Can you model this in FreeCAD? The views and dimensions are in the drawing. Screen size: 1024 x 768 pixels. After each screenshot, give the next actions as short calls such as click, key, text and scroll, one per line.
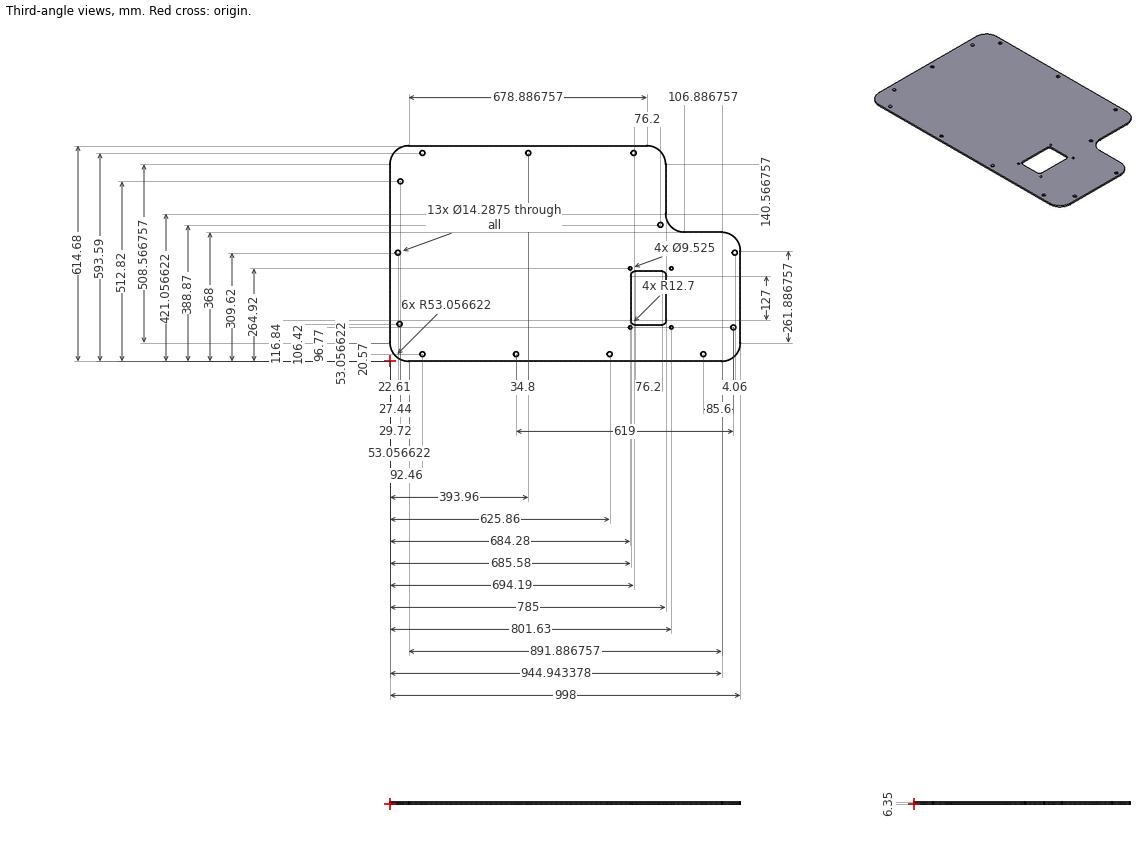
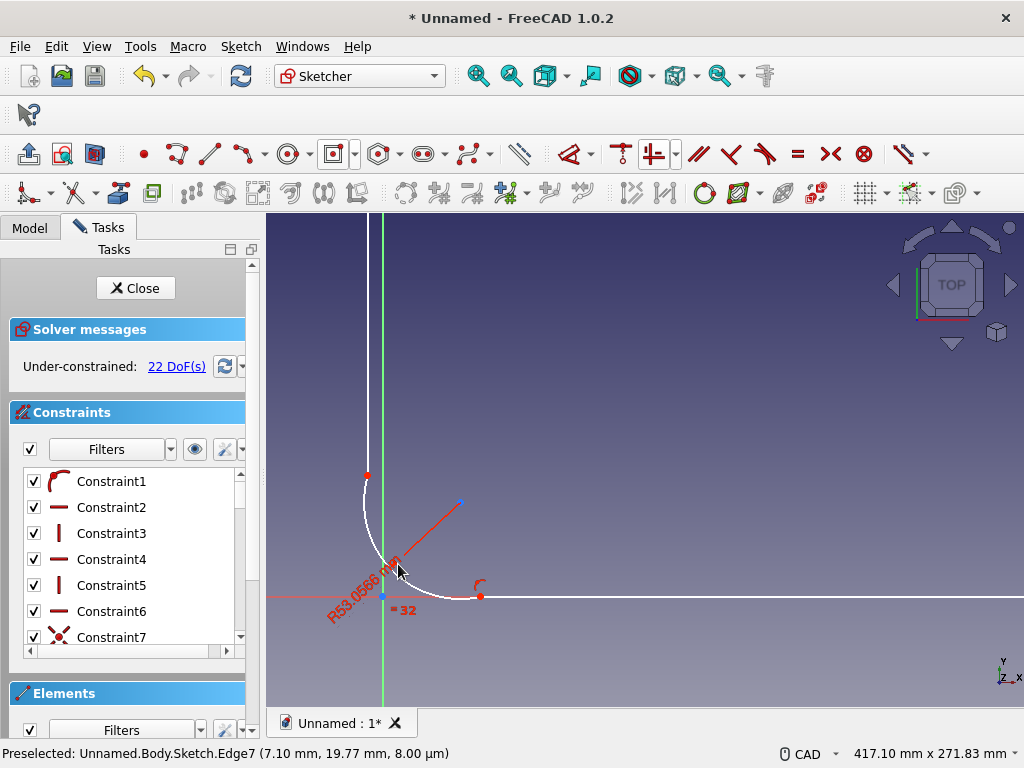
scroll(396, 567, down, 8)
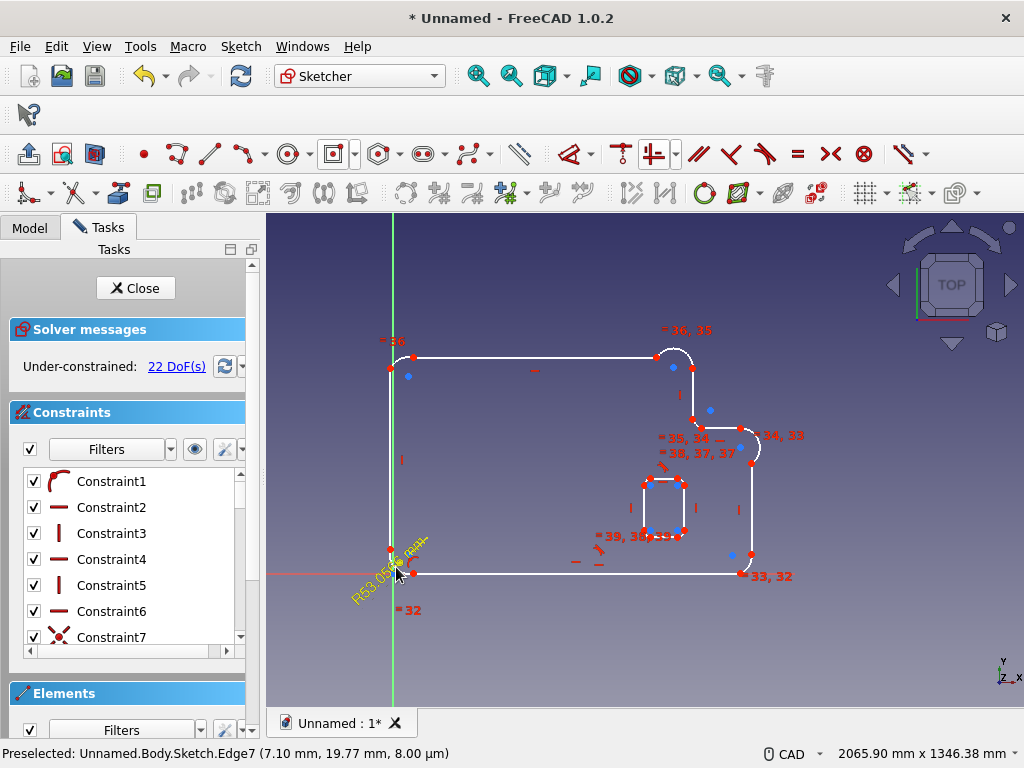
scroll(648, 479, up, 11)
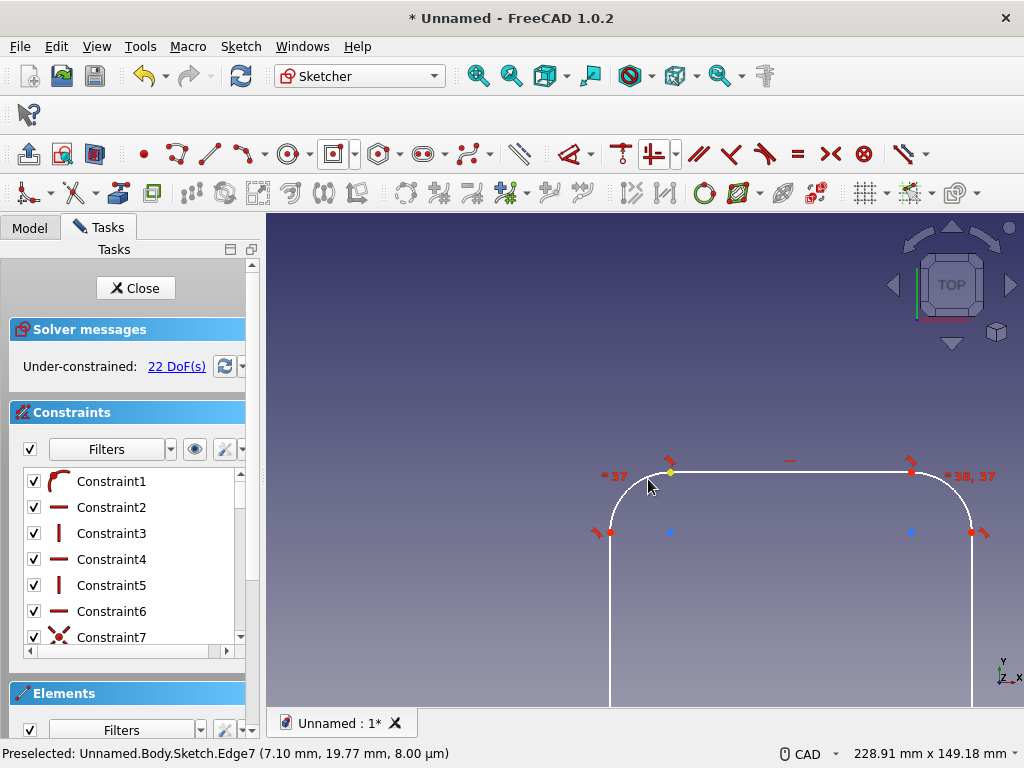
click(643, 479)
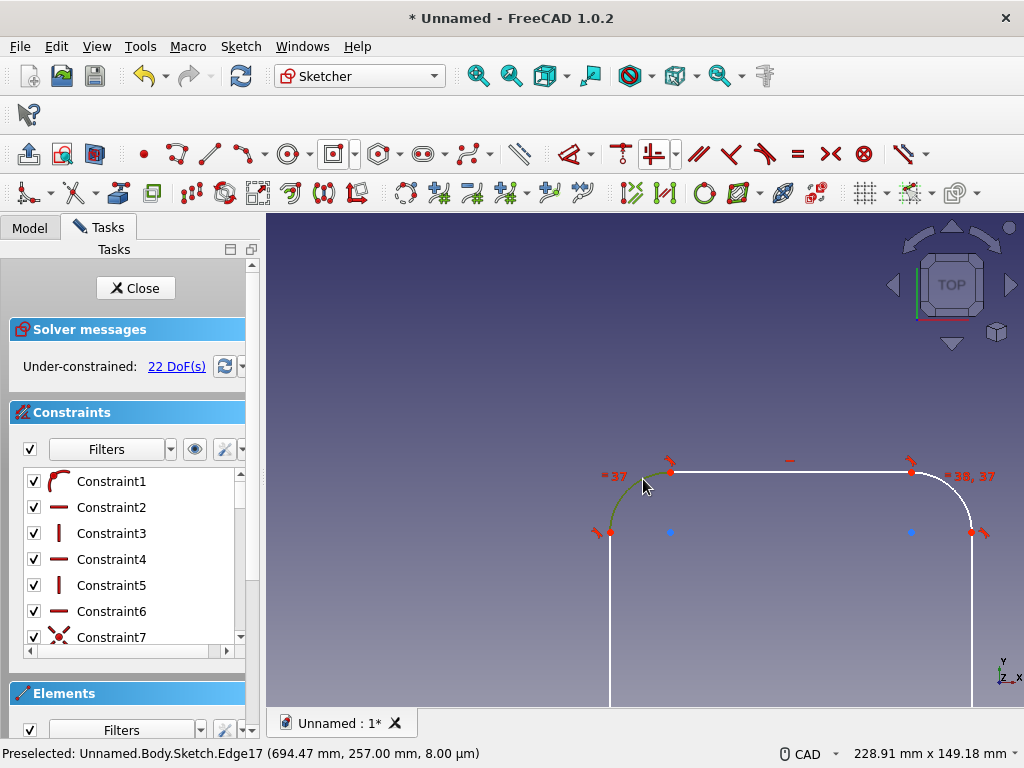
click(590, 154)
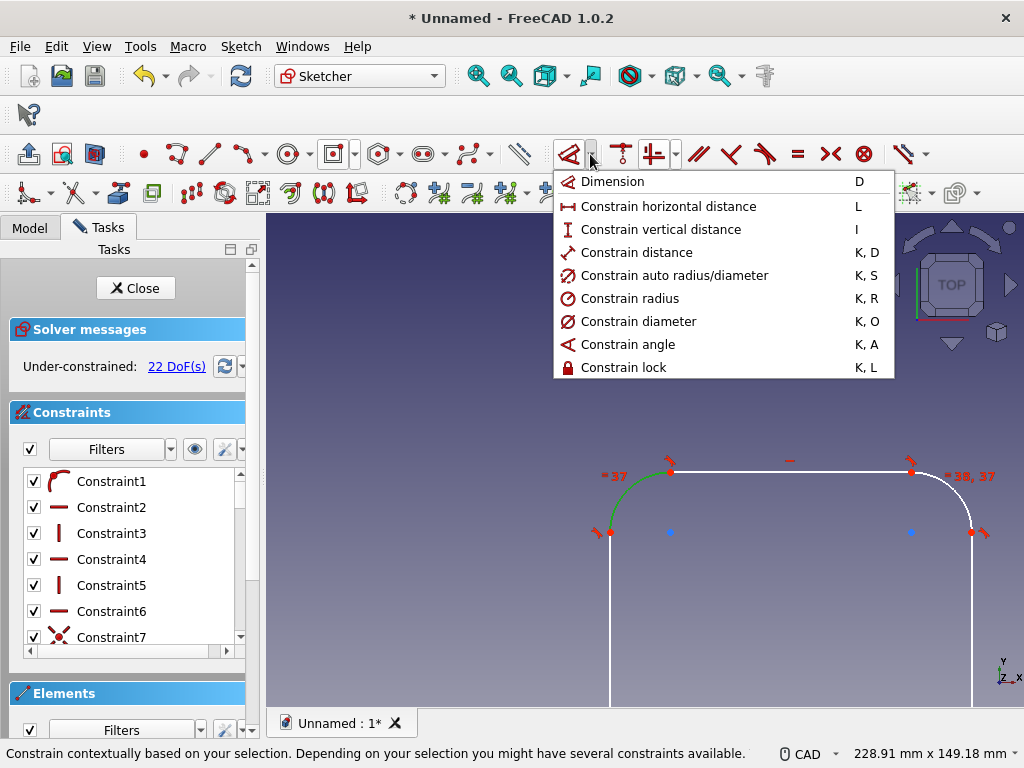
click(724, 298)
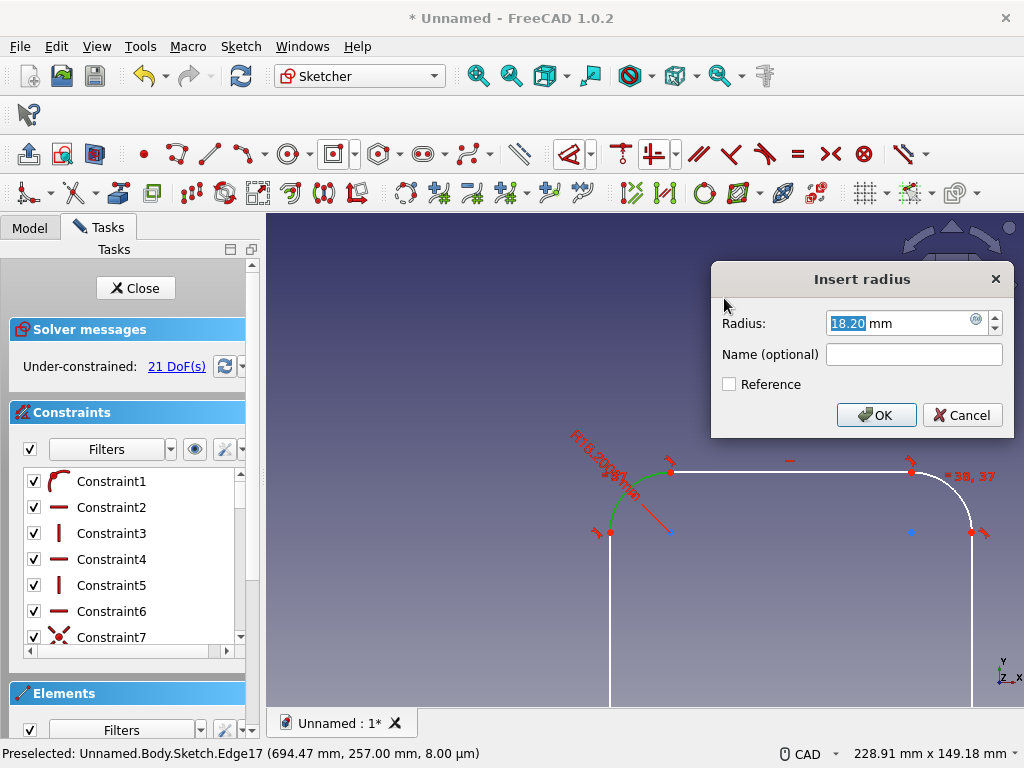
text(12.7)
key(Return)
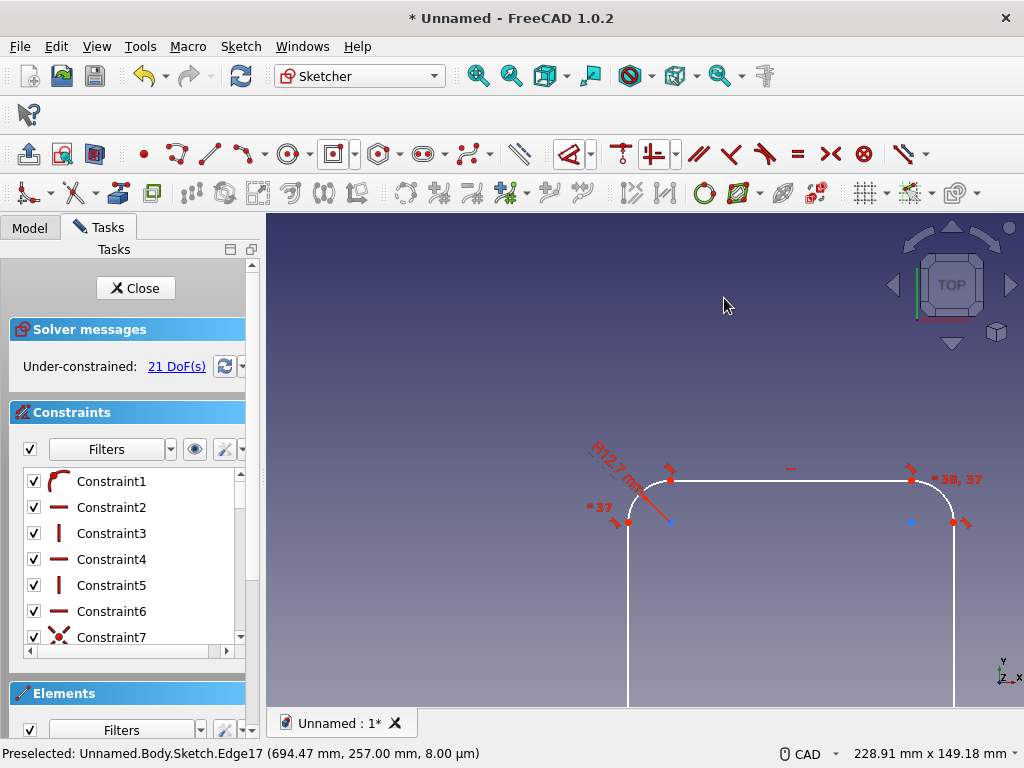
scroll(648, 479, down, 11)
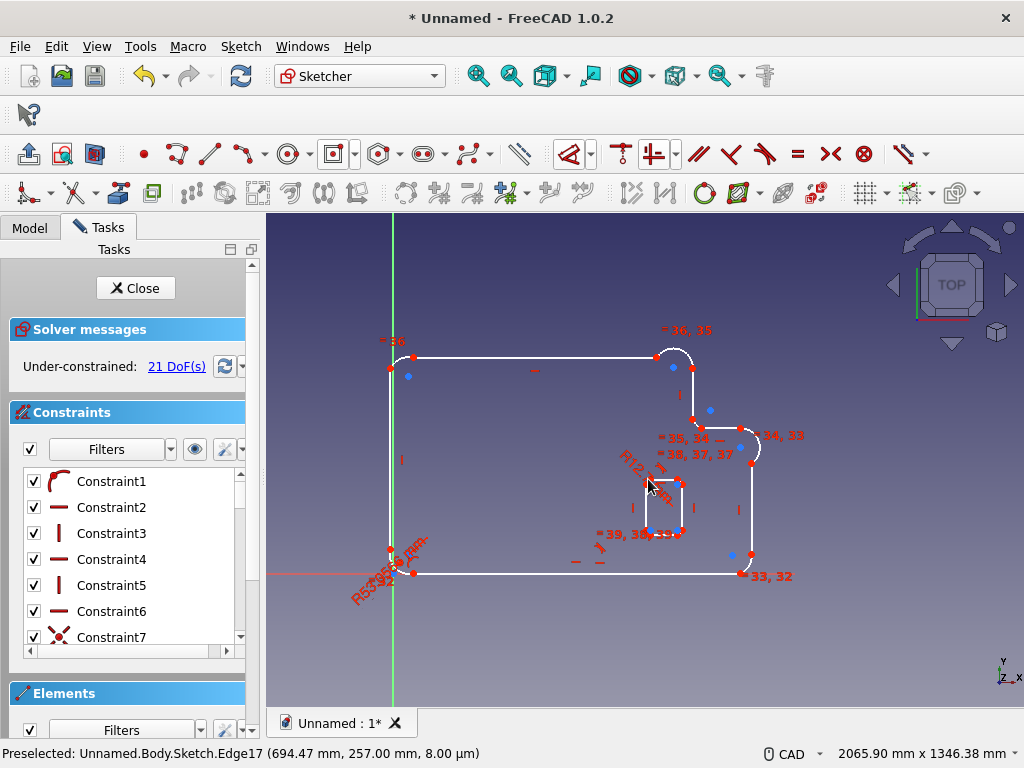
click(390, 369)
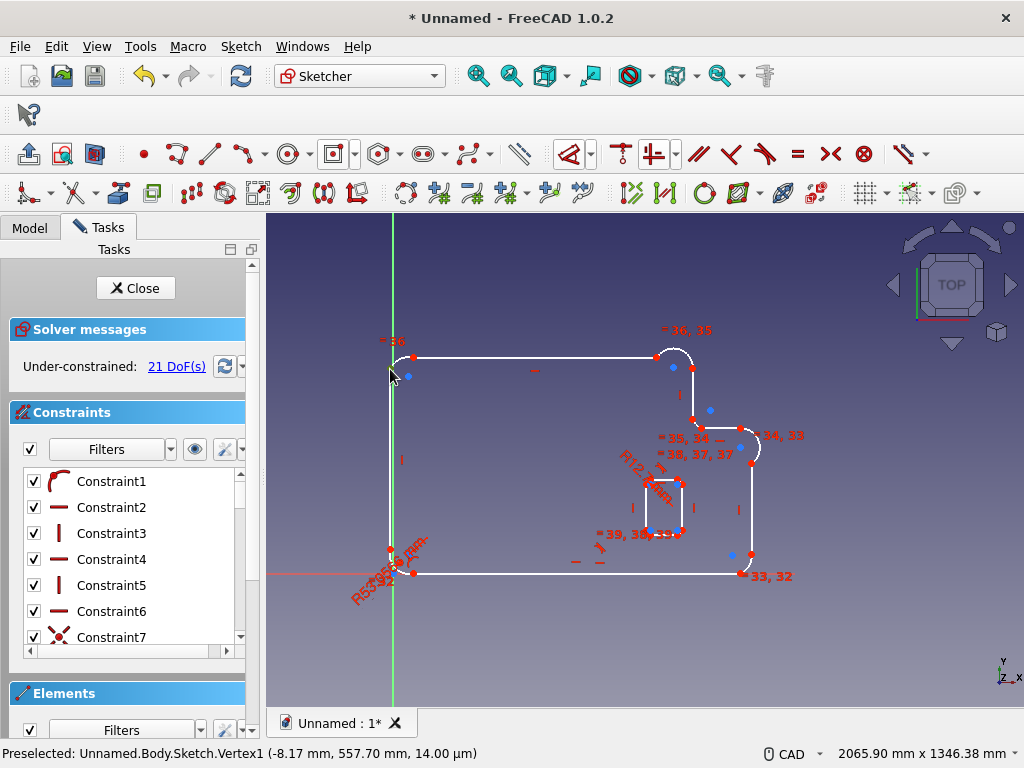
click(393, 648)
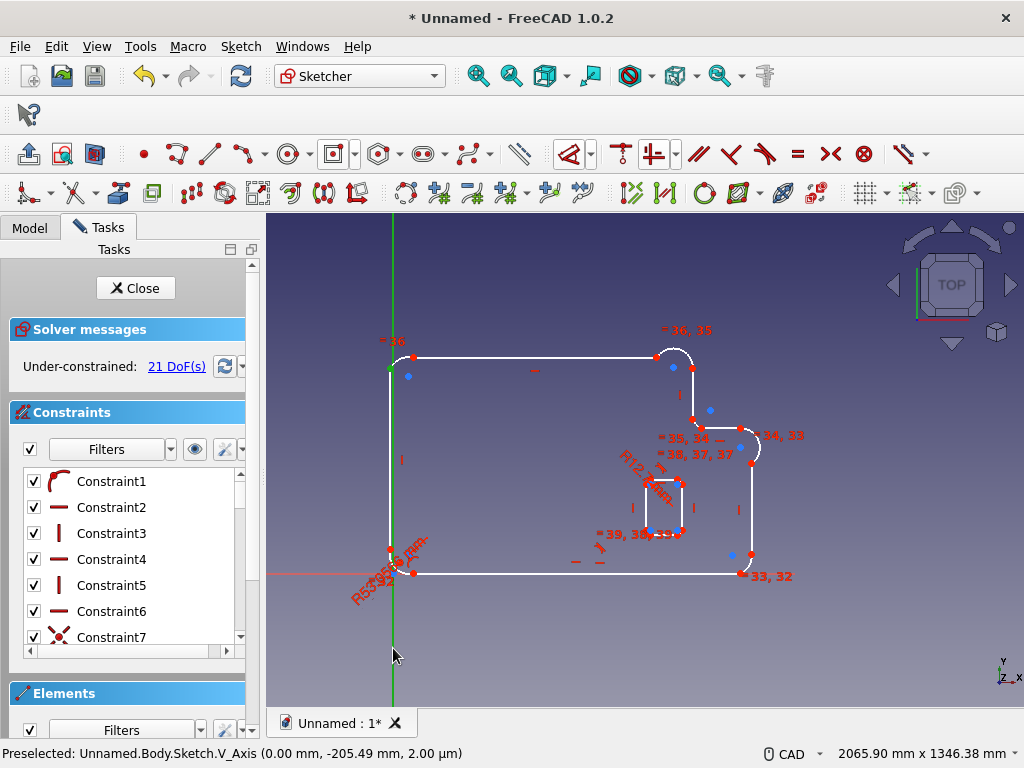
click(621, 154)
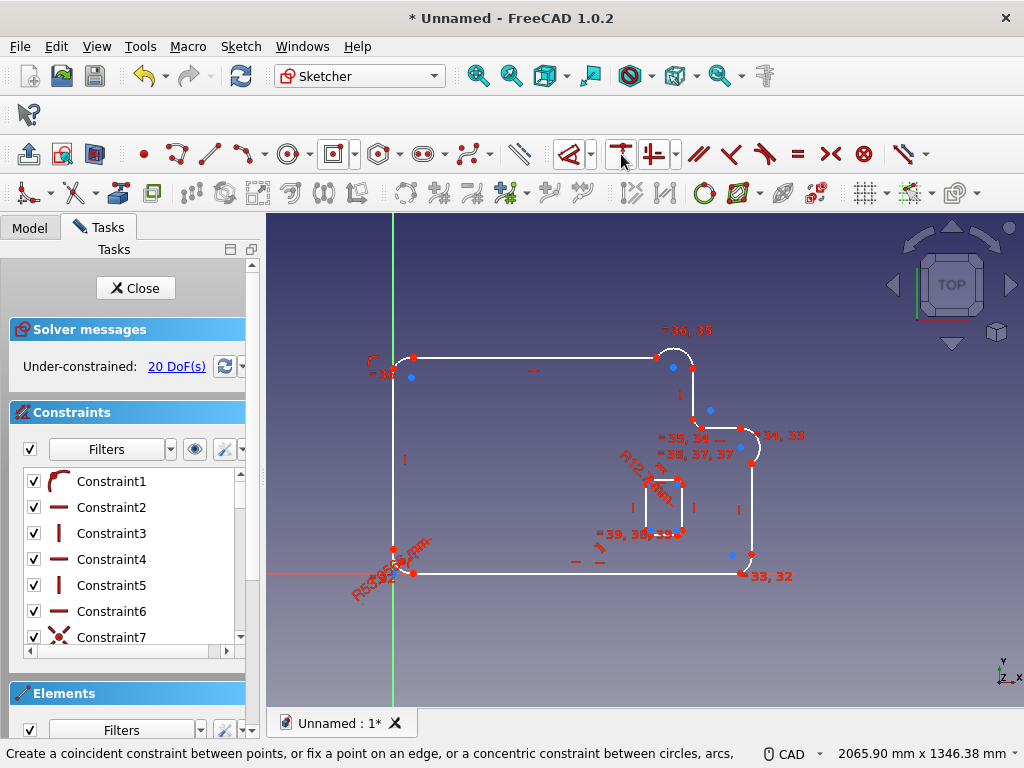
click(646, 517)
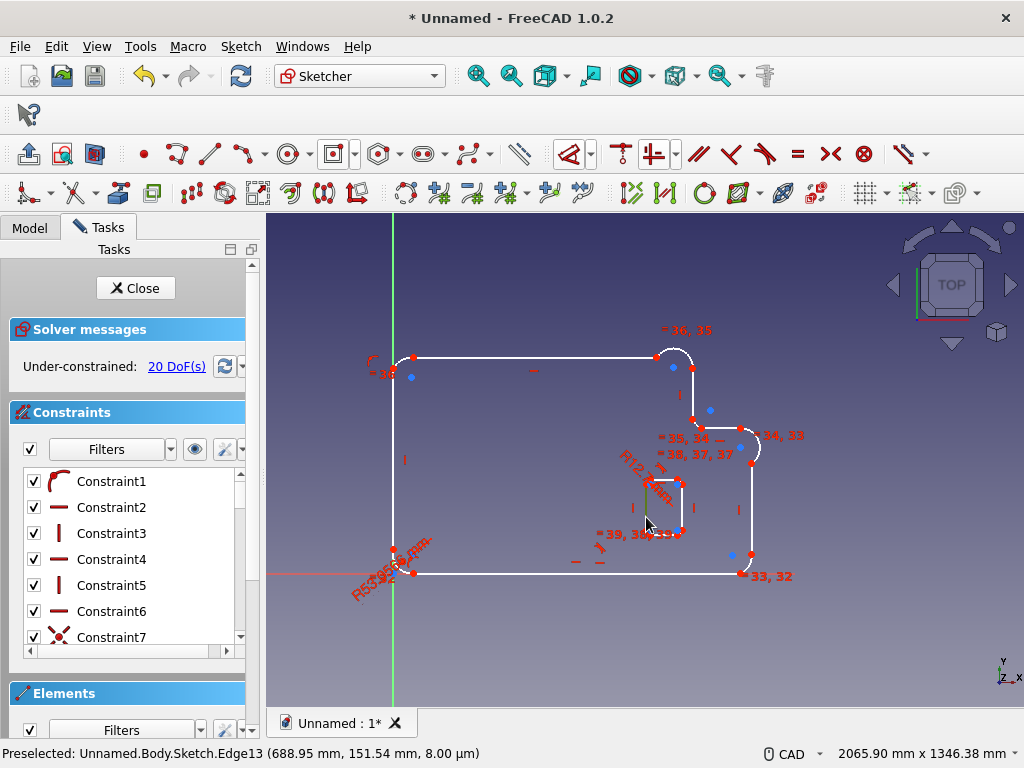
key(i)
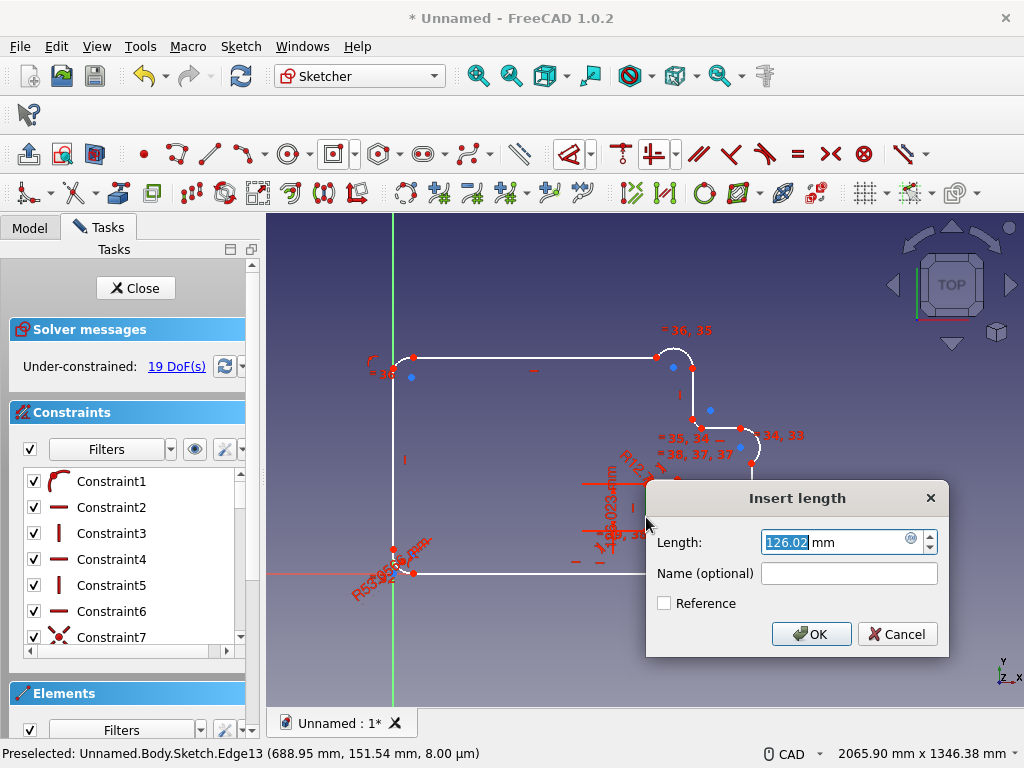
text(127)
key(Return)